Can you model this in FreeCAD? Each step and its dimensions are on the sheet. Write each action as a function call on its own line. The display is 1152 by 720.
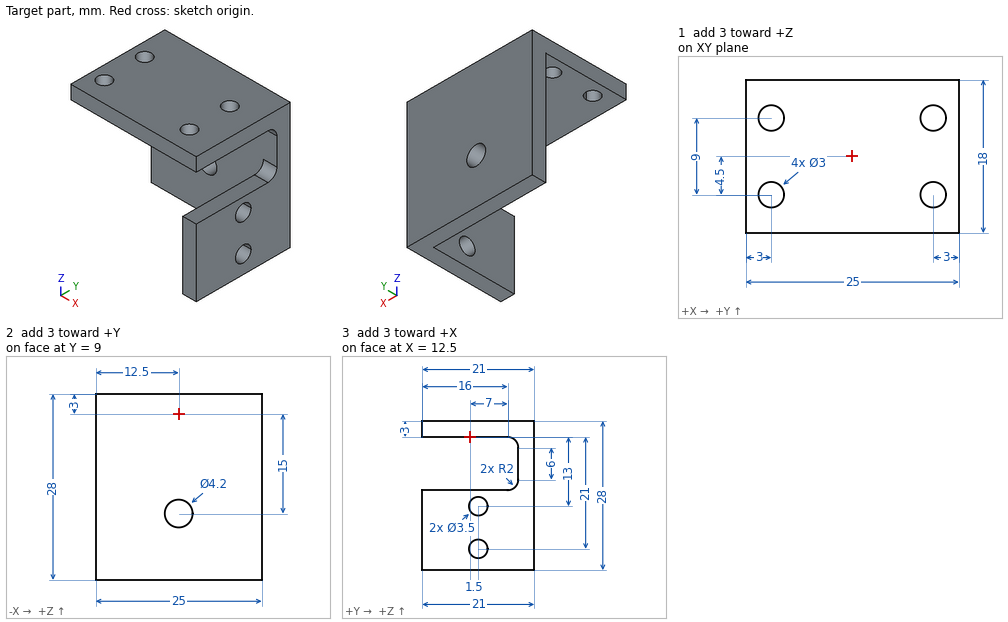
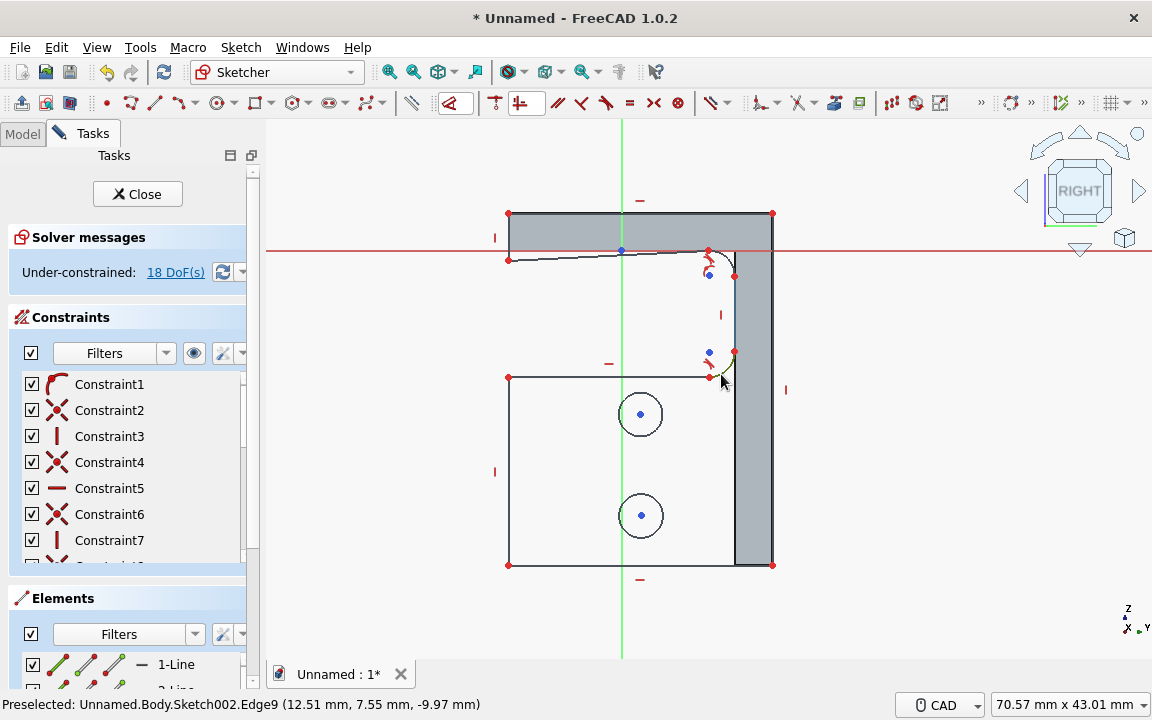
key(t)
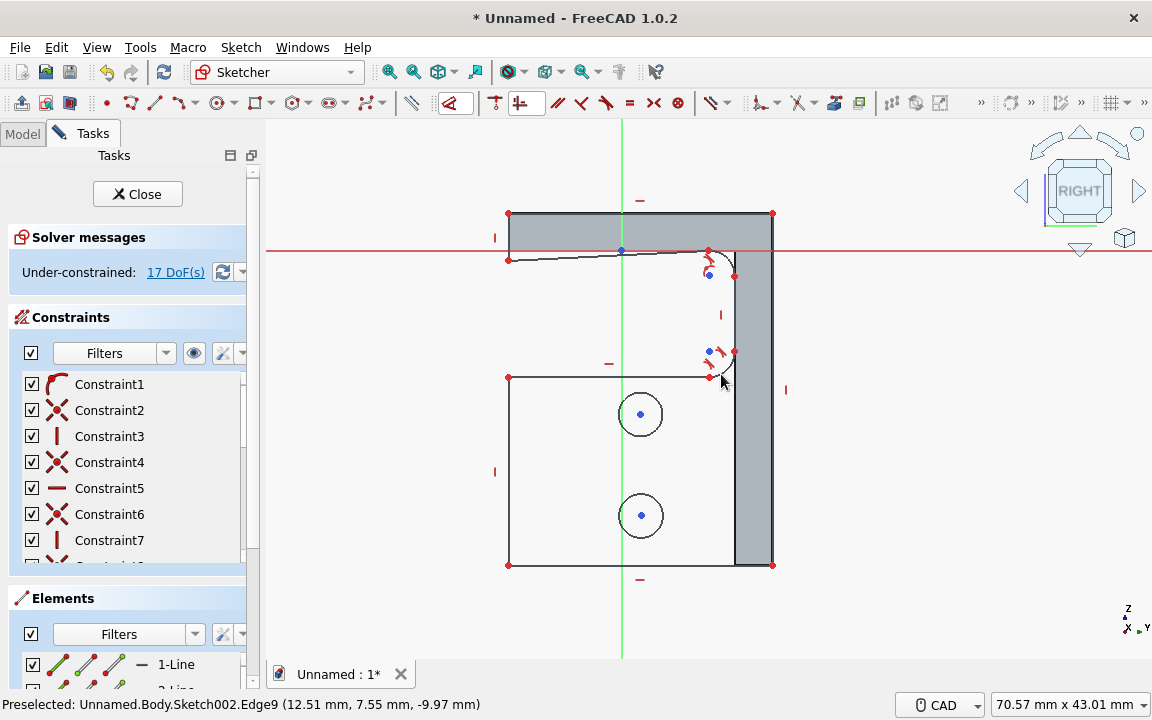
click(735, 330)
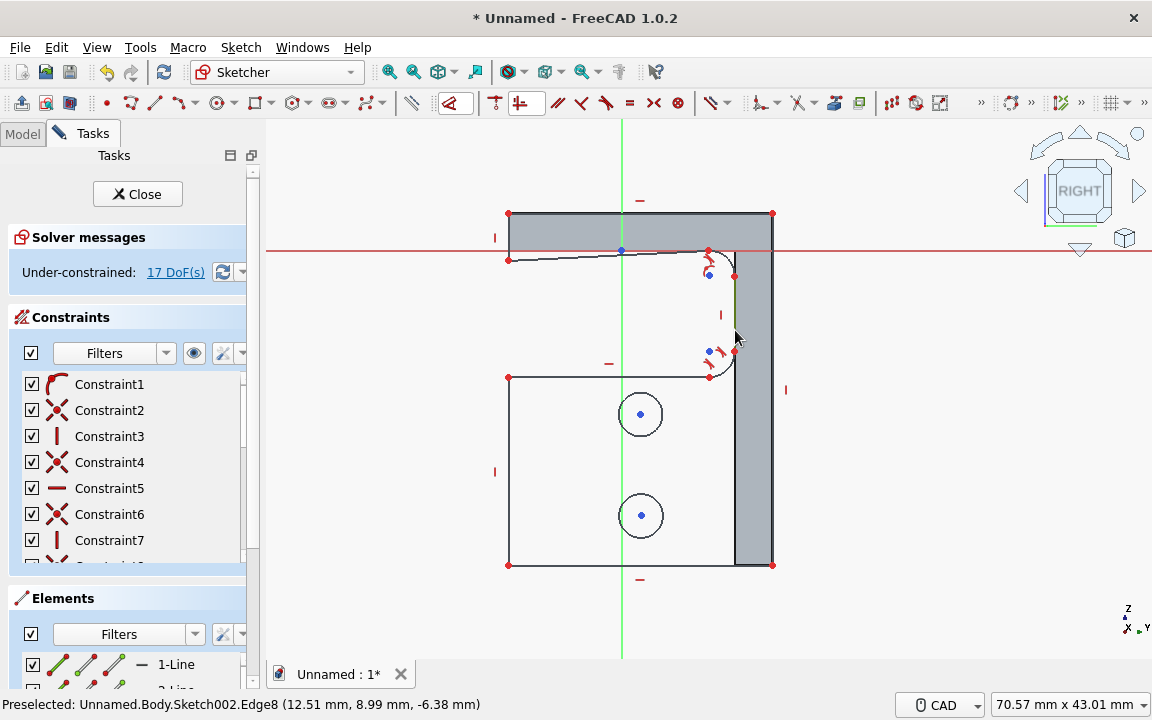
click(732, 265)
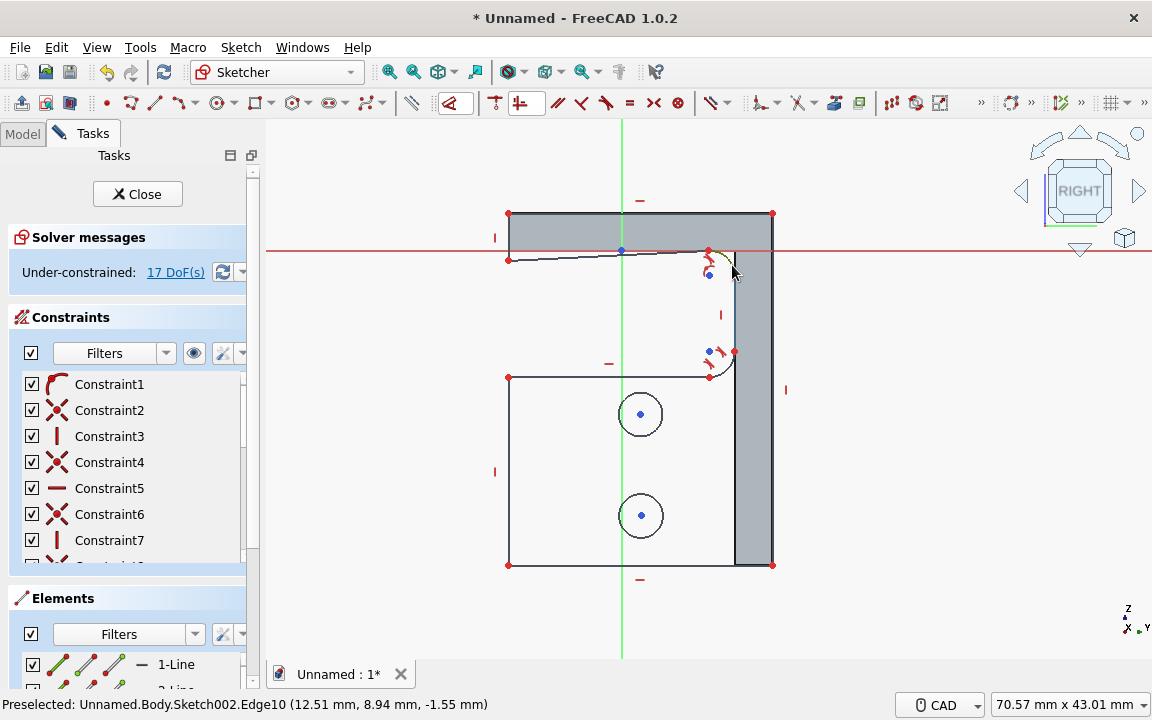
key(t)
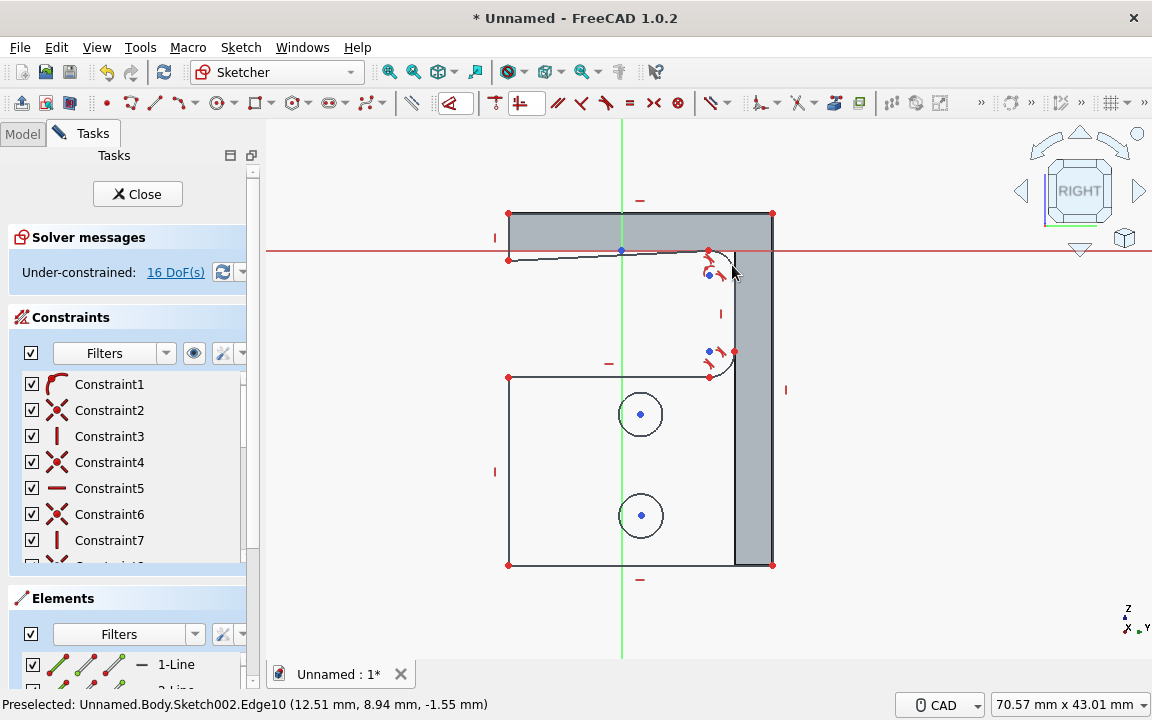
click(649, 254)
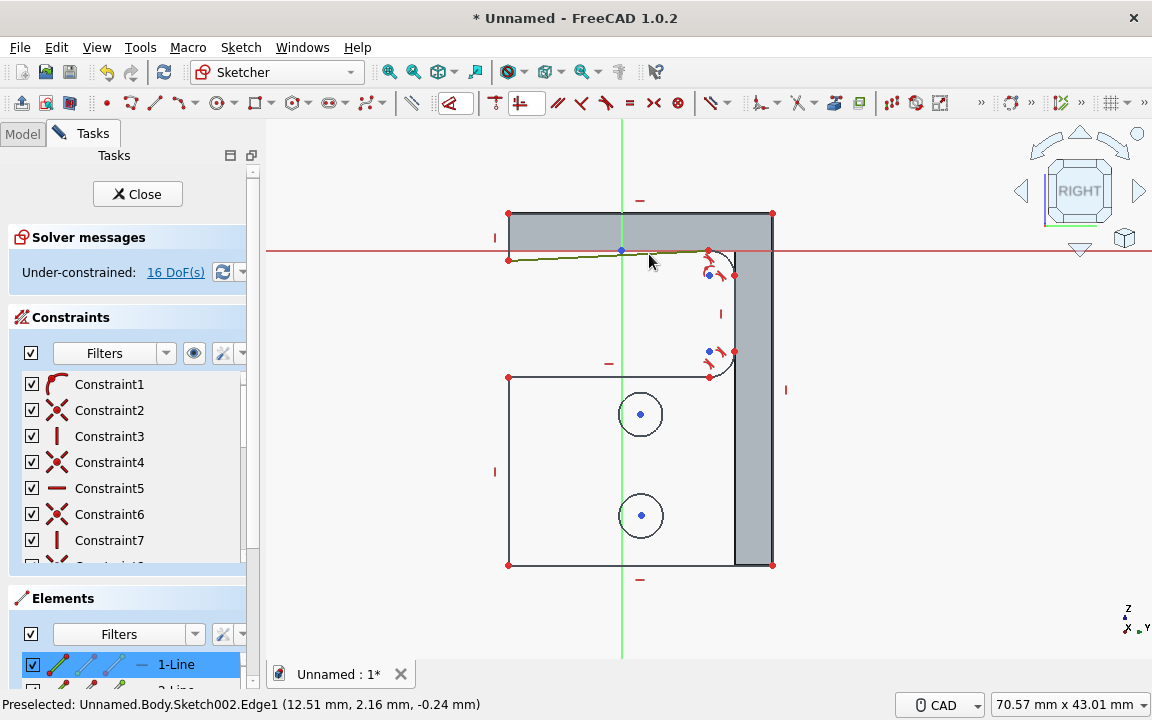
key(h)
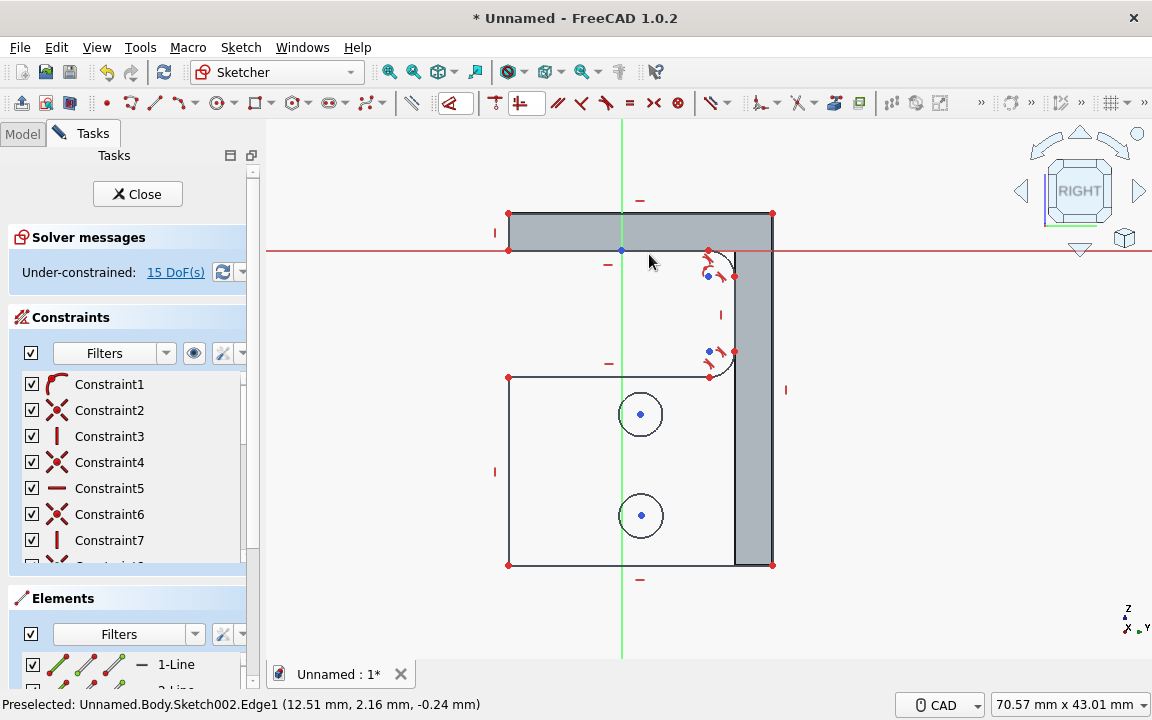
click(721, 374)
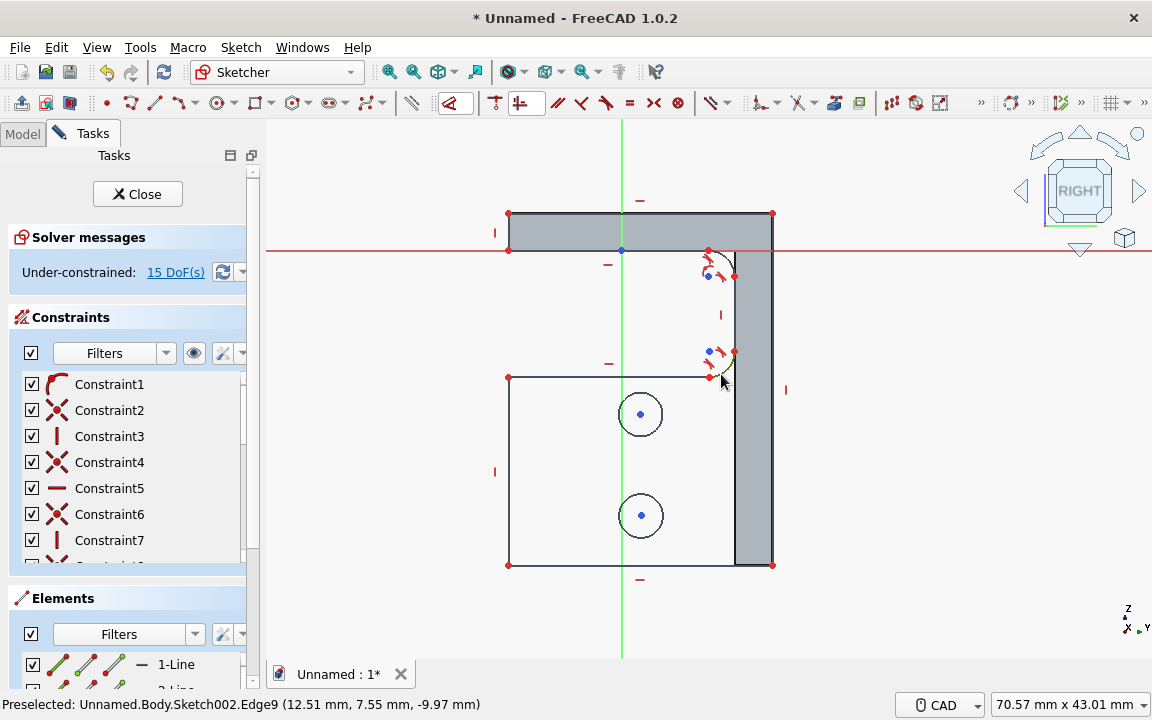
click(732, 265)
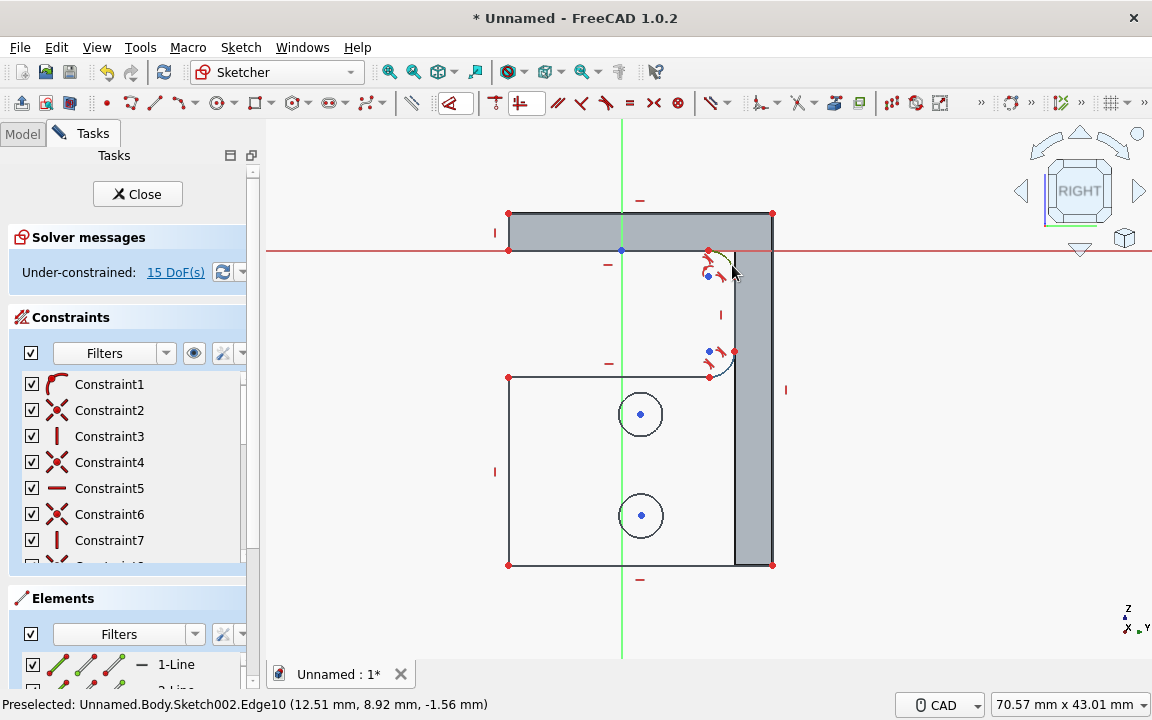
key(e)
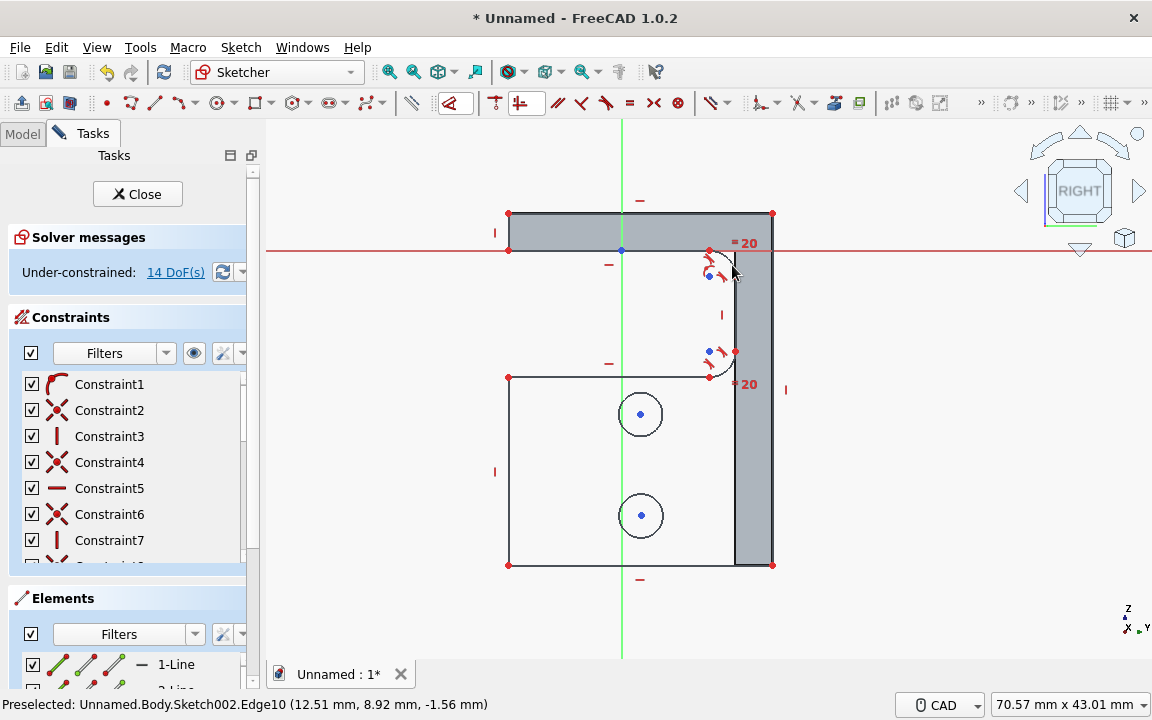
click(656, 399)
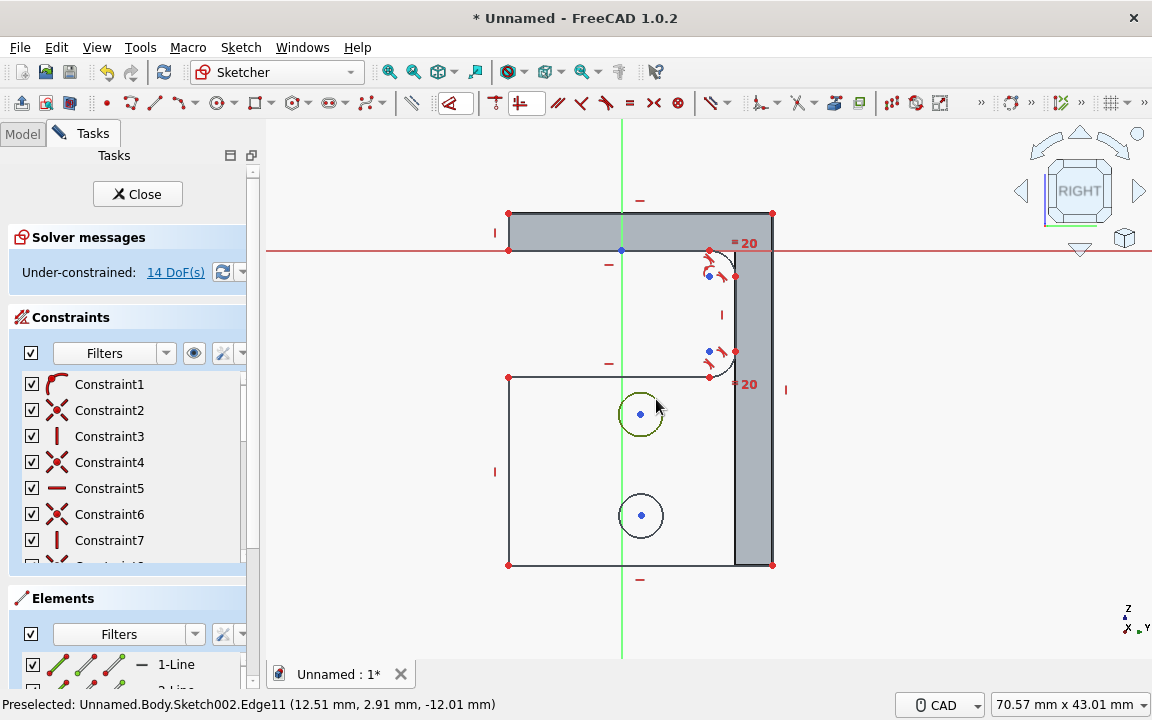
click(656, 500)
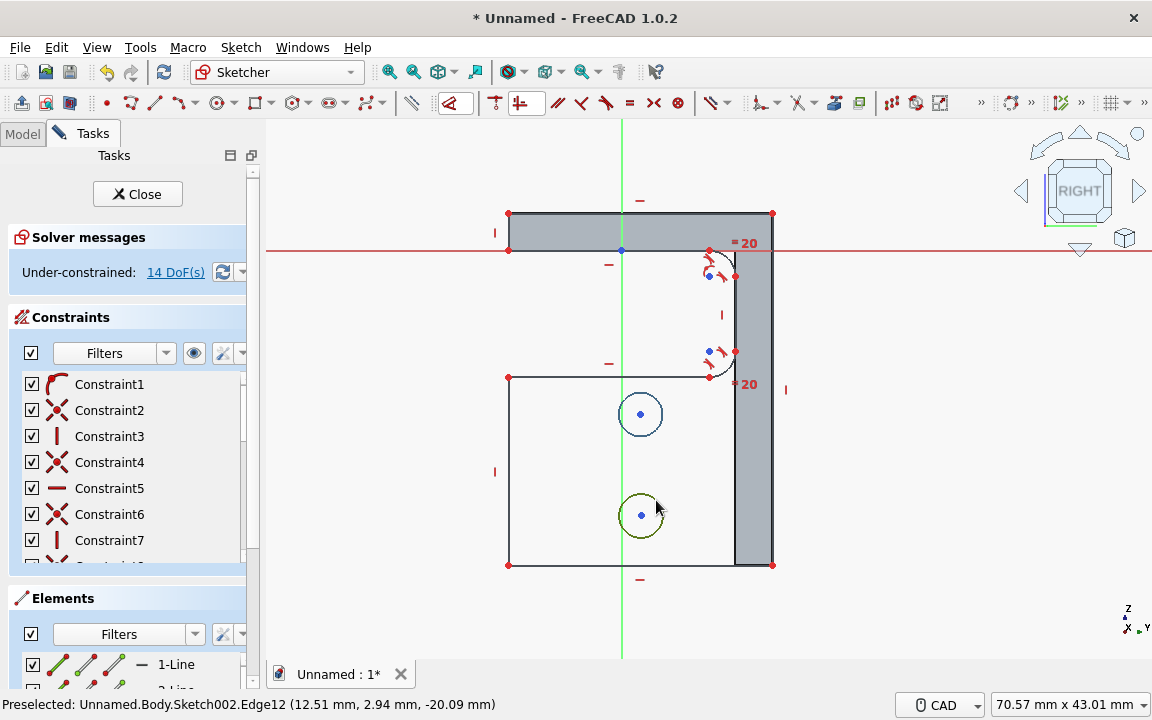
key(e)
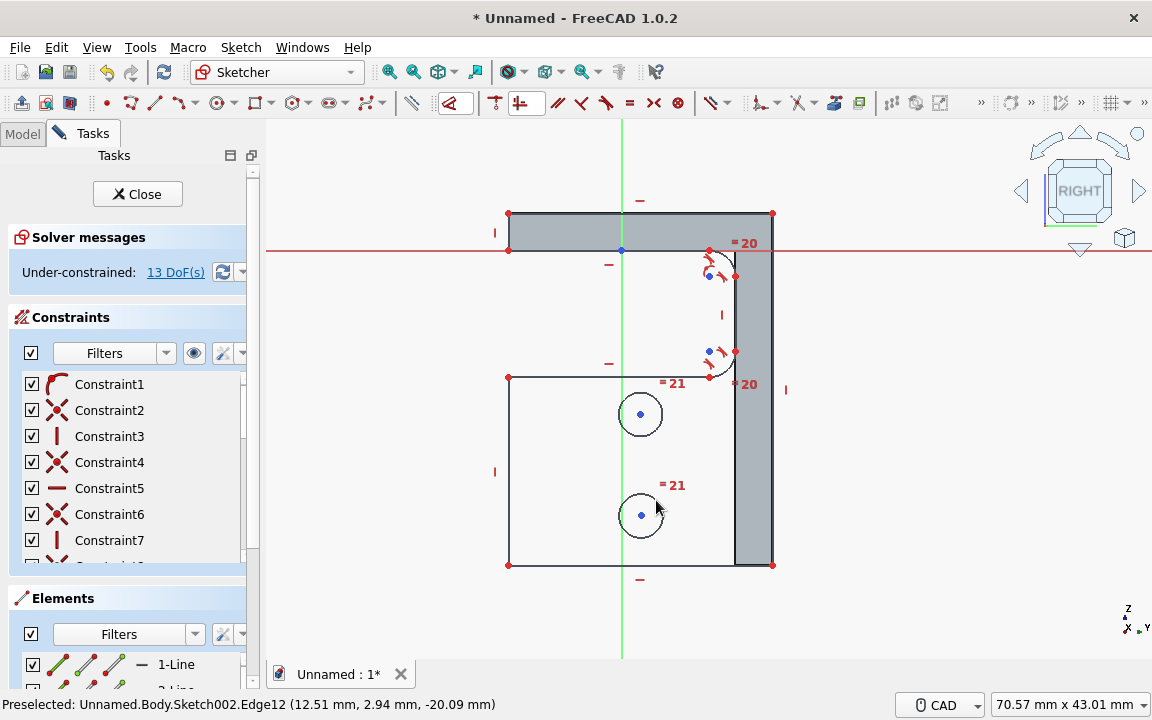
click(641, 415)